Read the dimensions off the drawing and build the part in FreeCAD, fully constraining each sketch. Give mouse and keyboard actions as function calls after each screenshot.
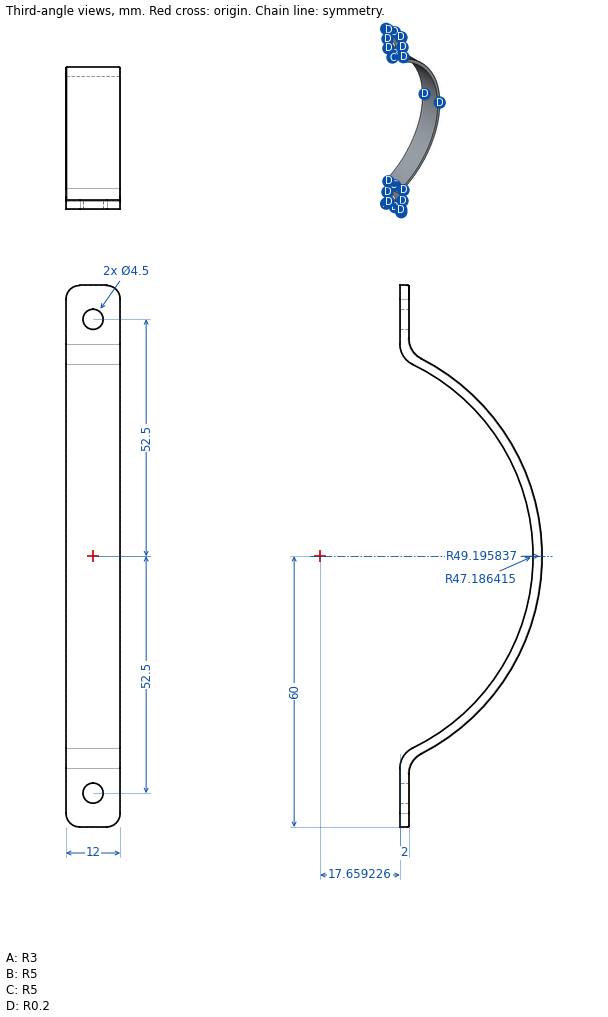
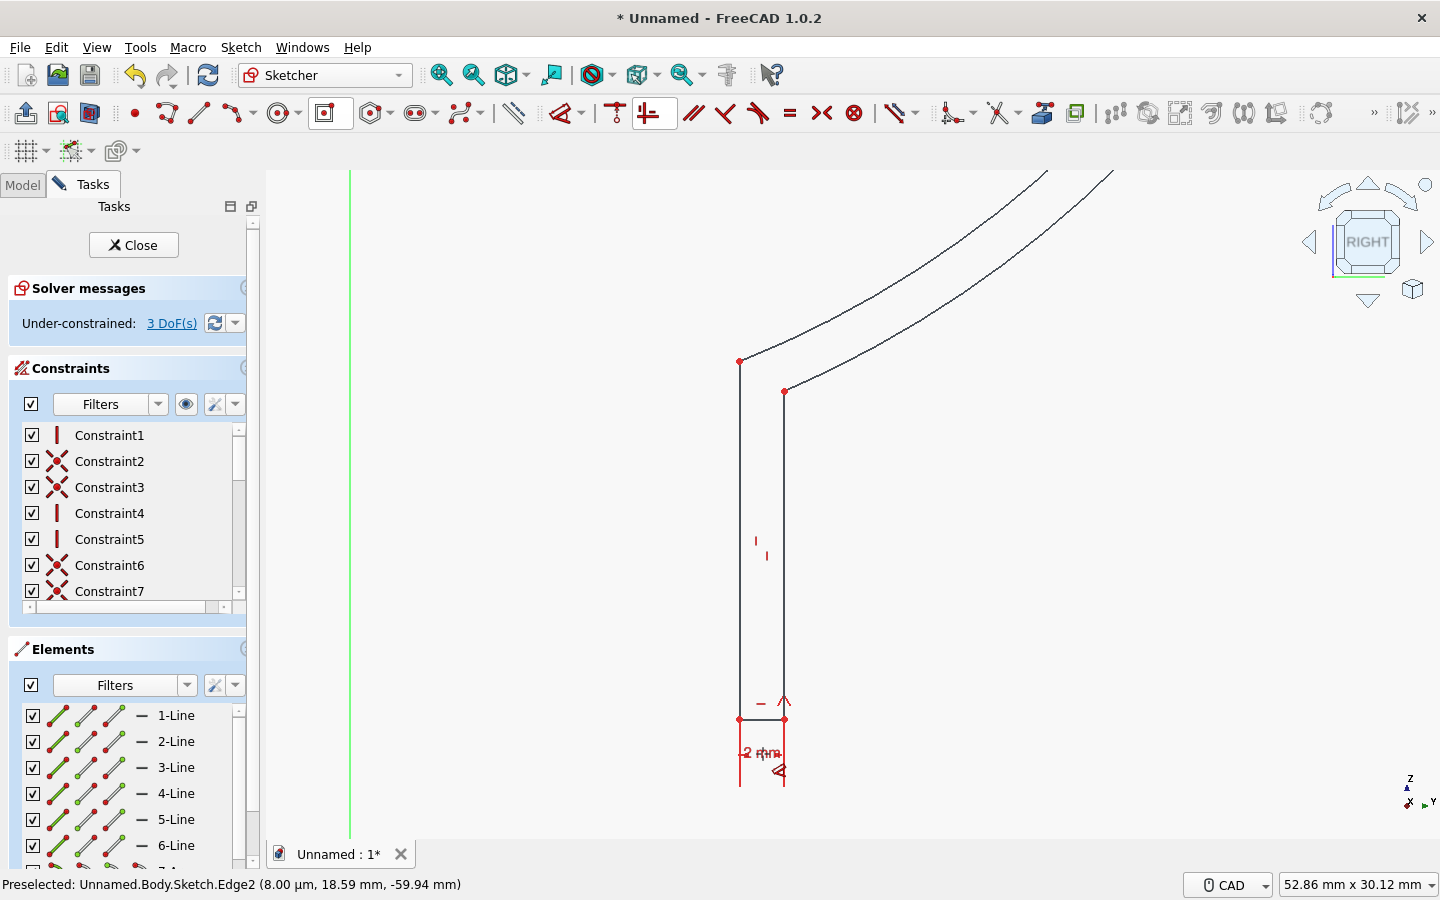
scroll(762, 725, down, 9)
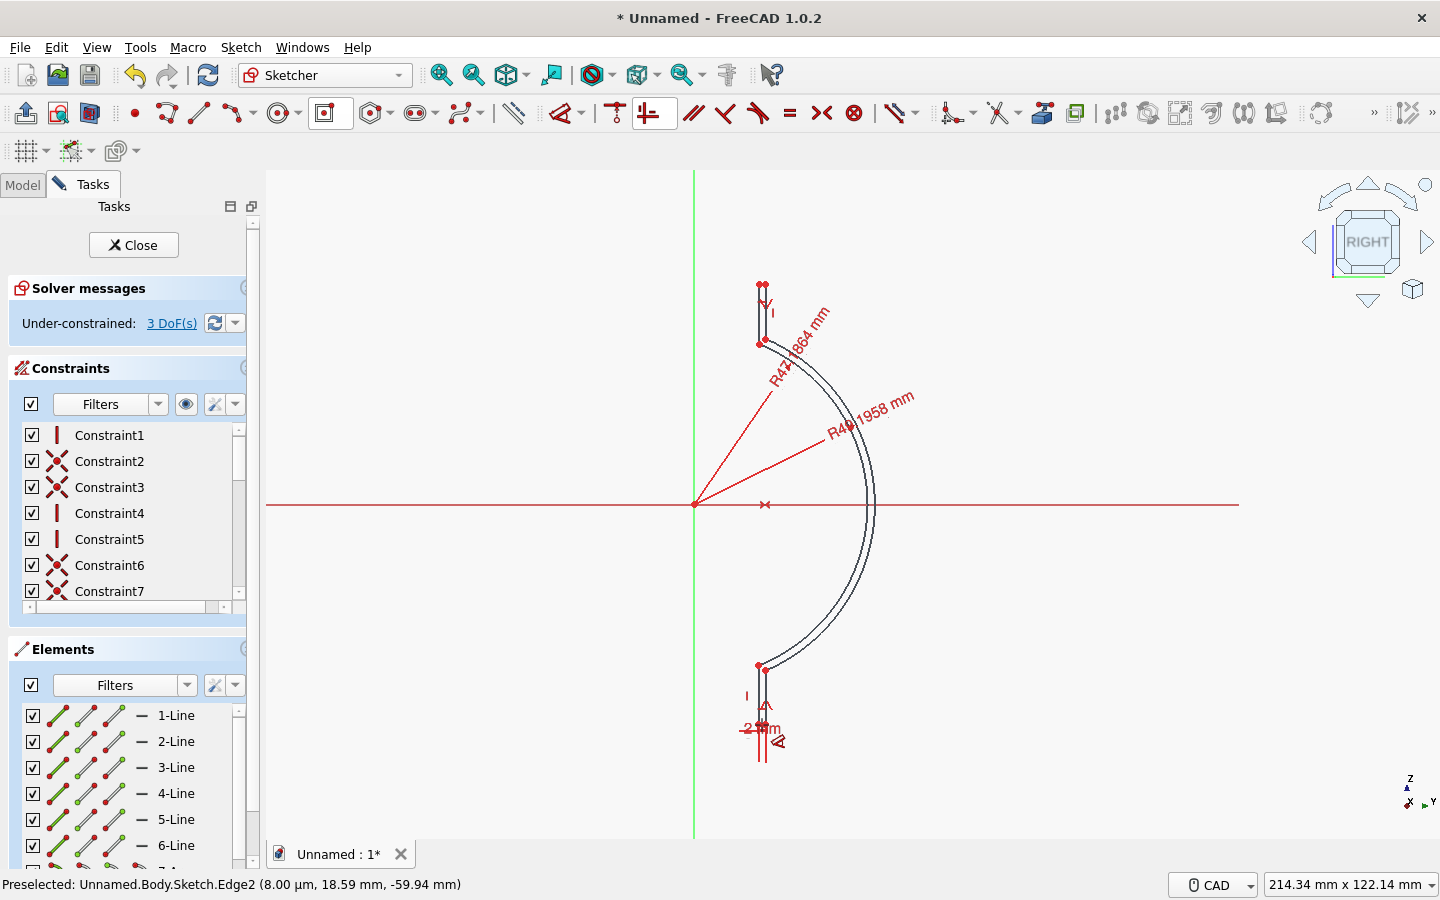
scroll(764, 285, up, 10)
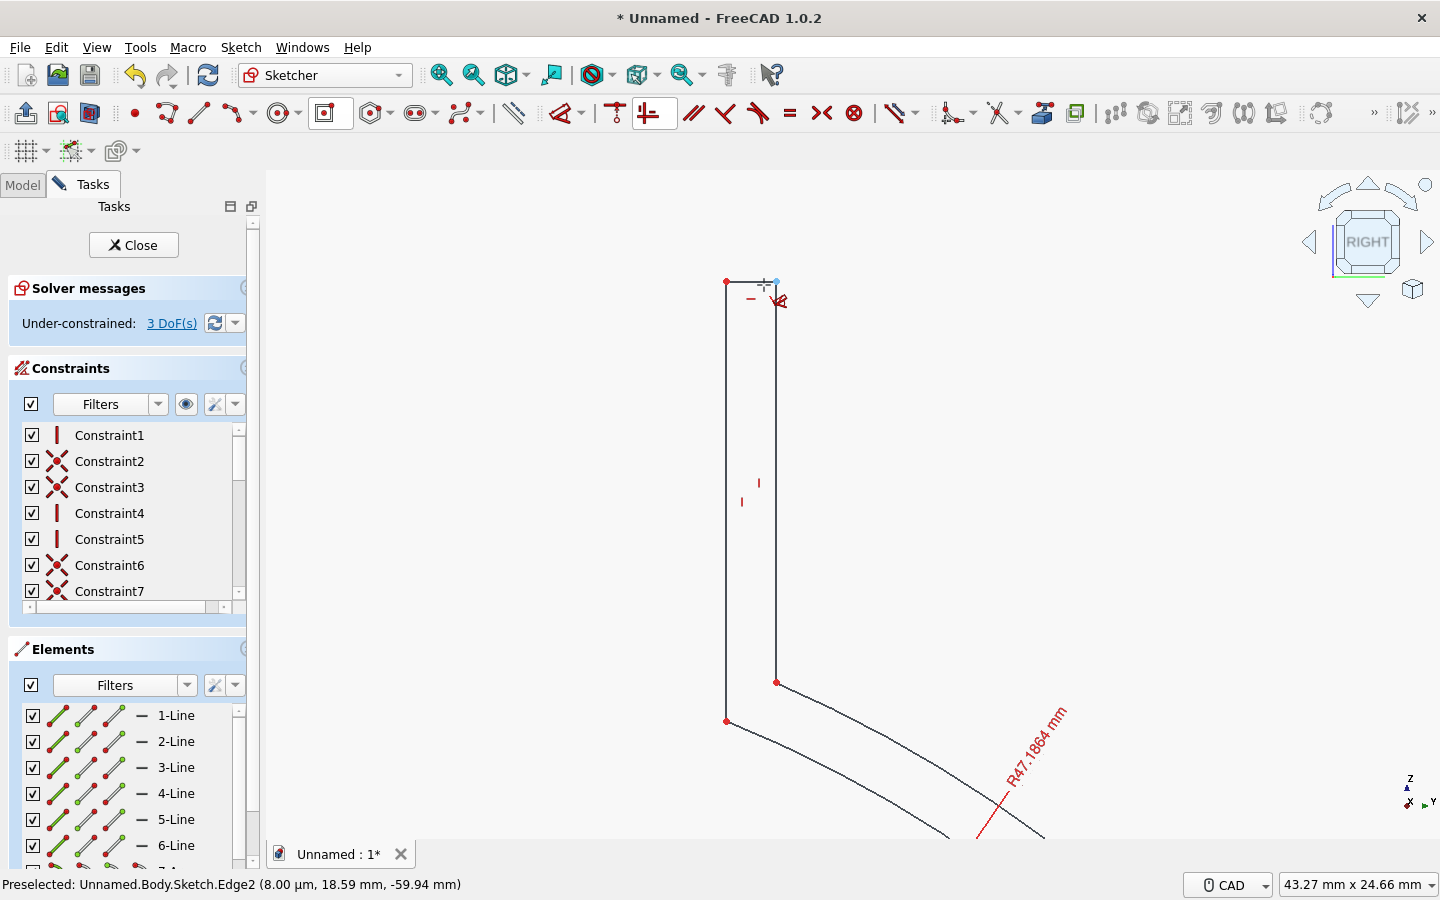
click(761, 282)
click(751, 248)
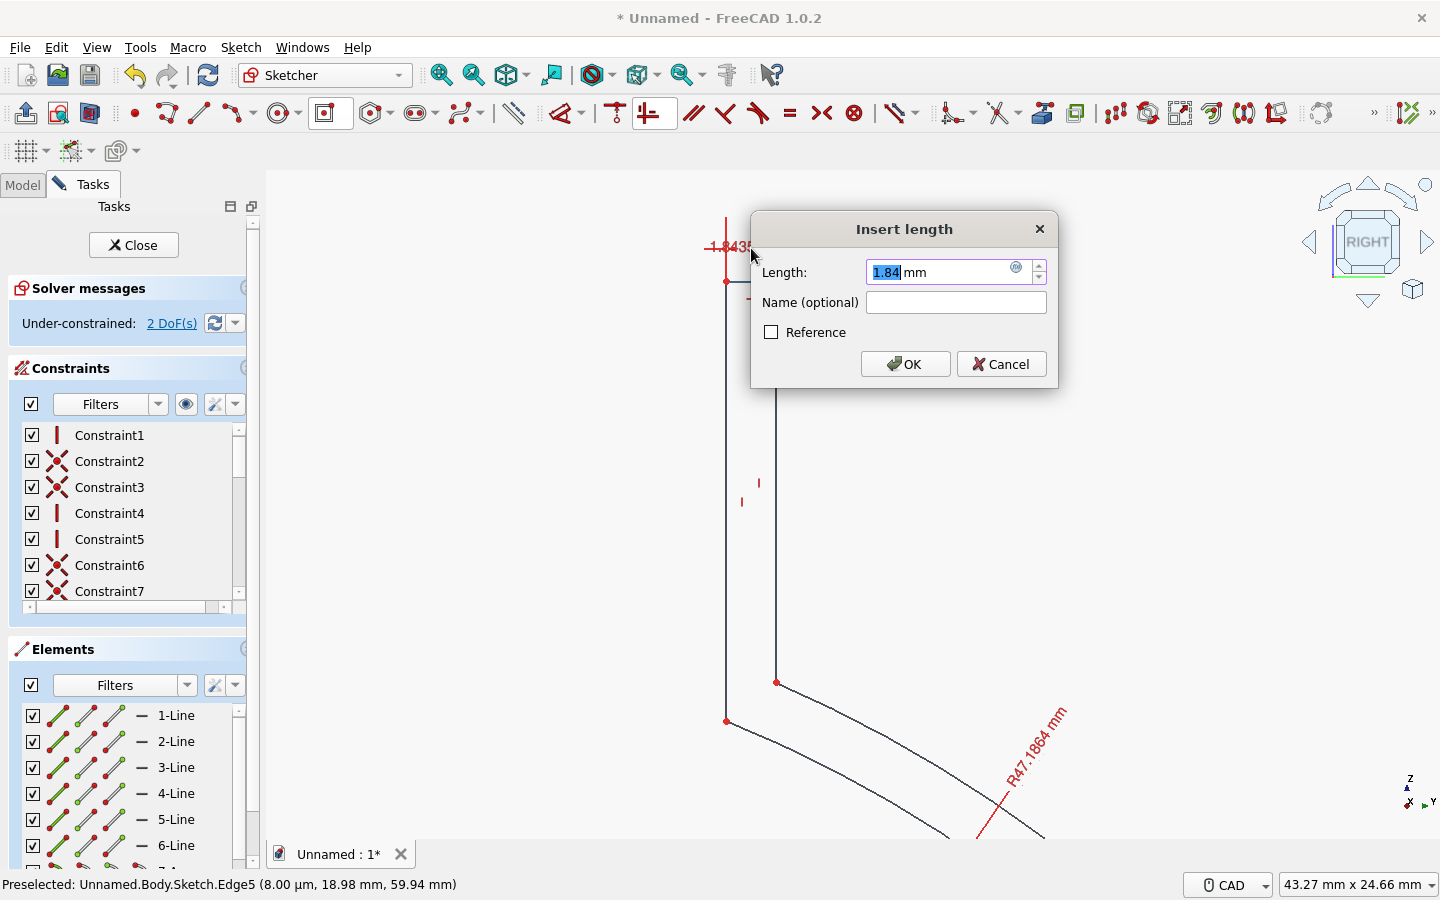
text(2)
key(Return)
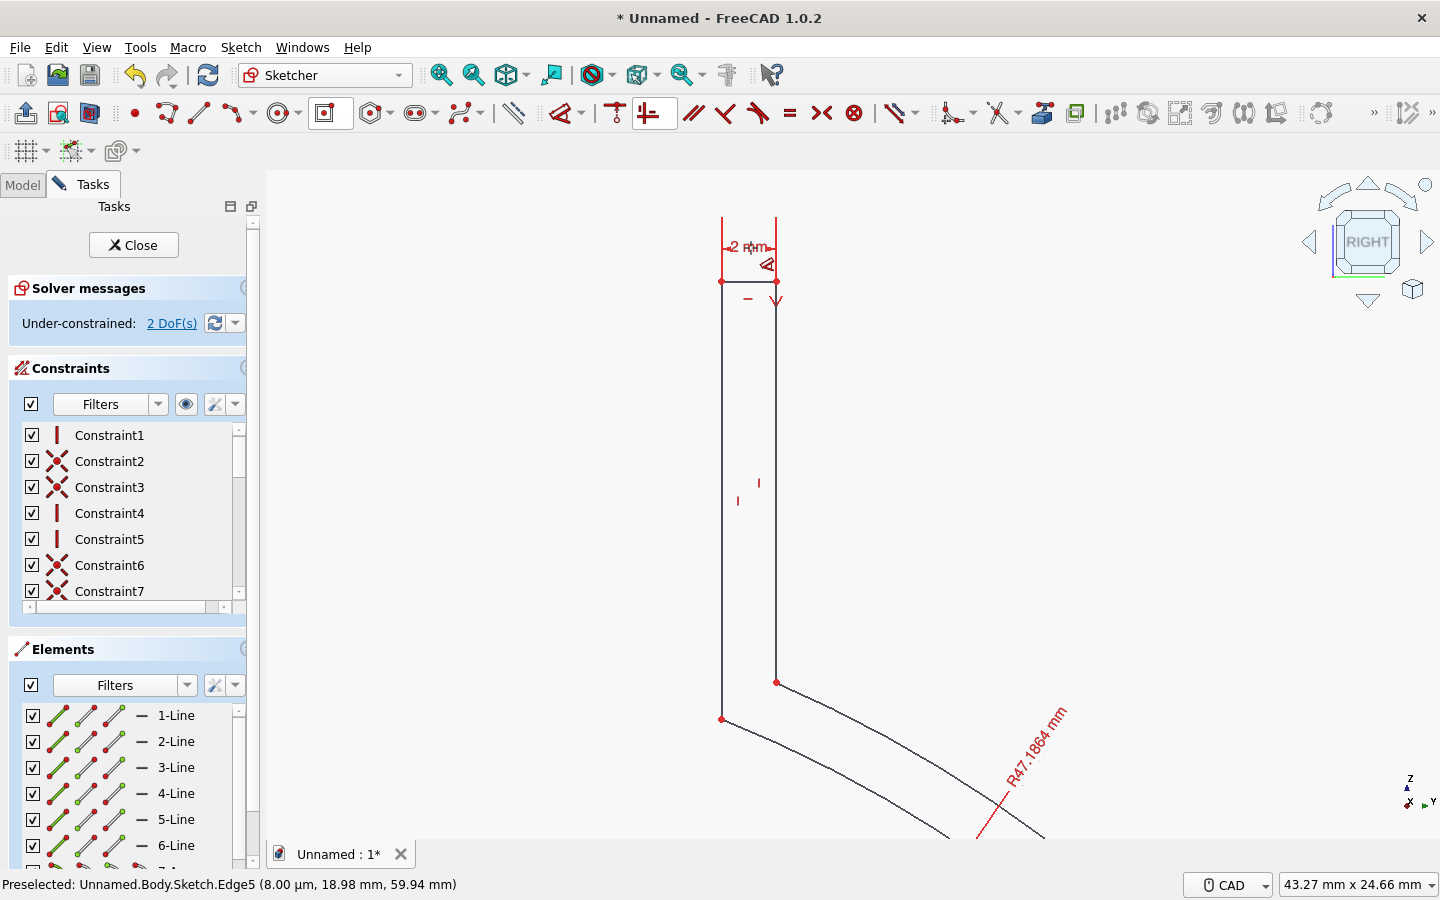
scroll(764, 285, down, 10)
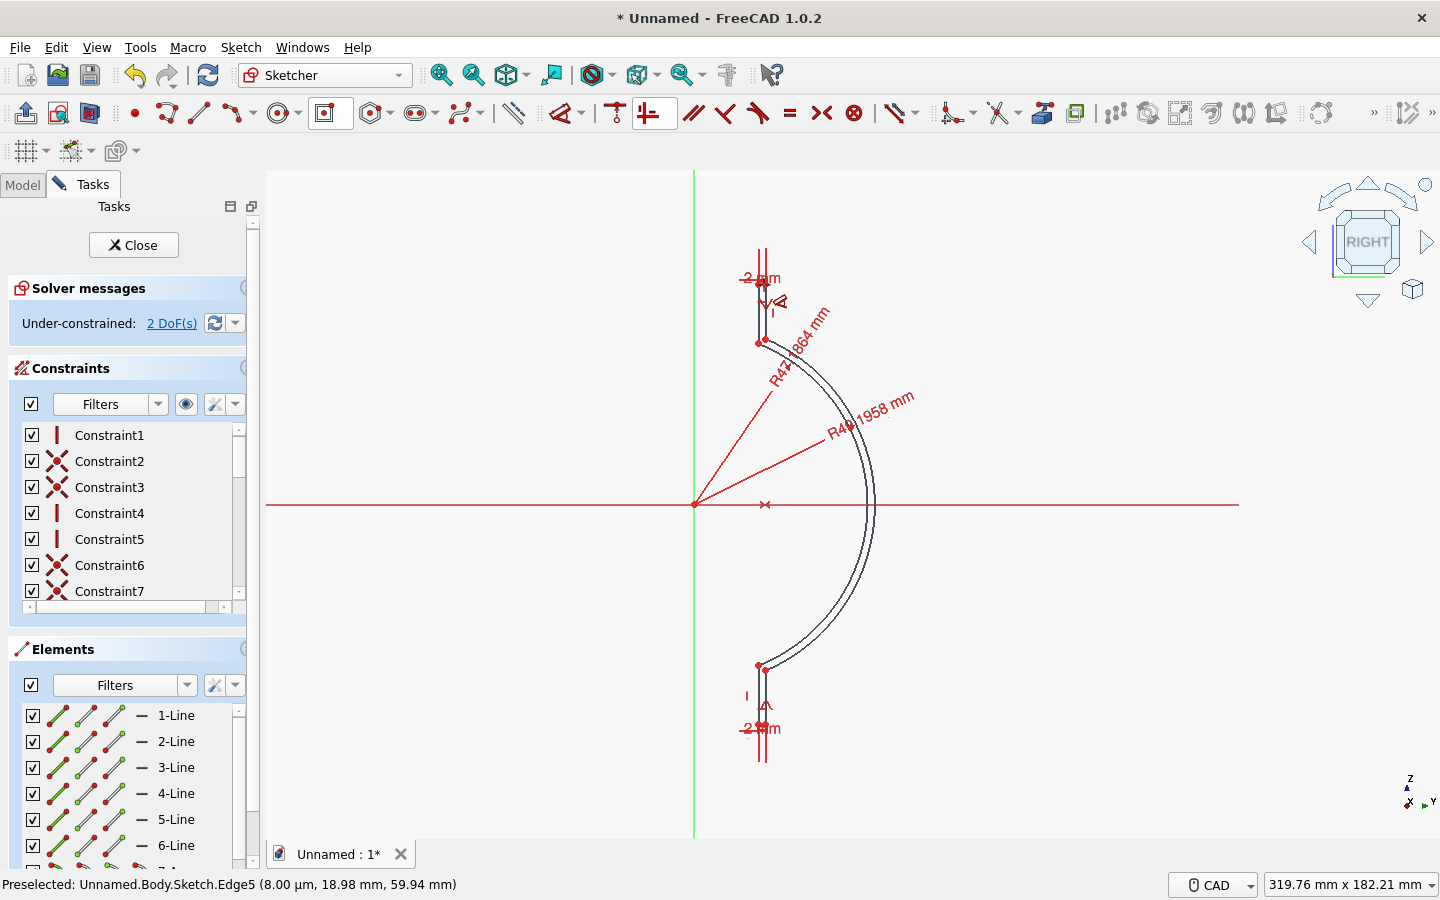
scroll(759, 725, up, 3)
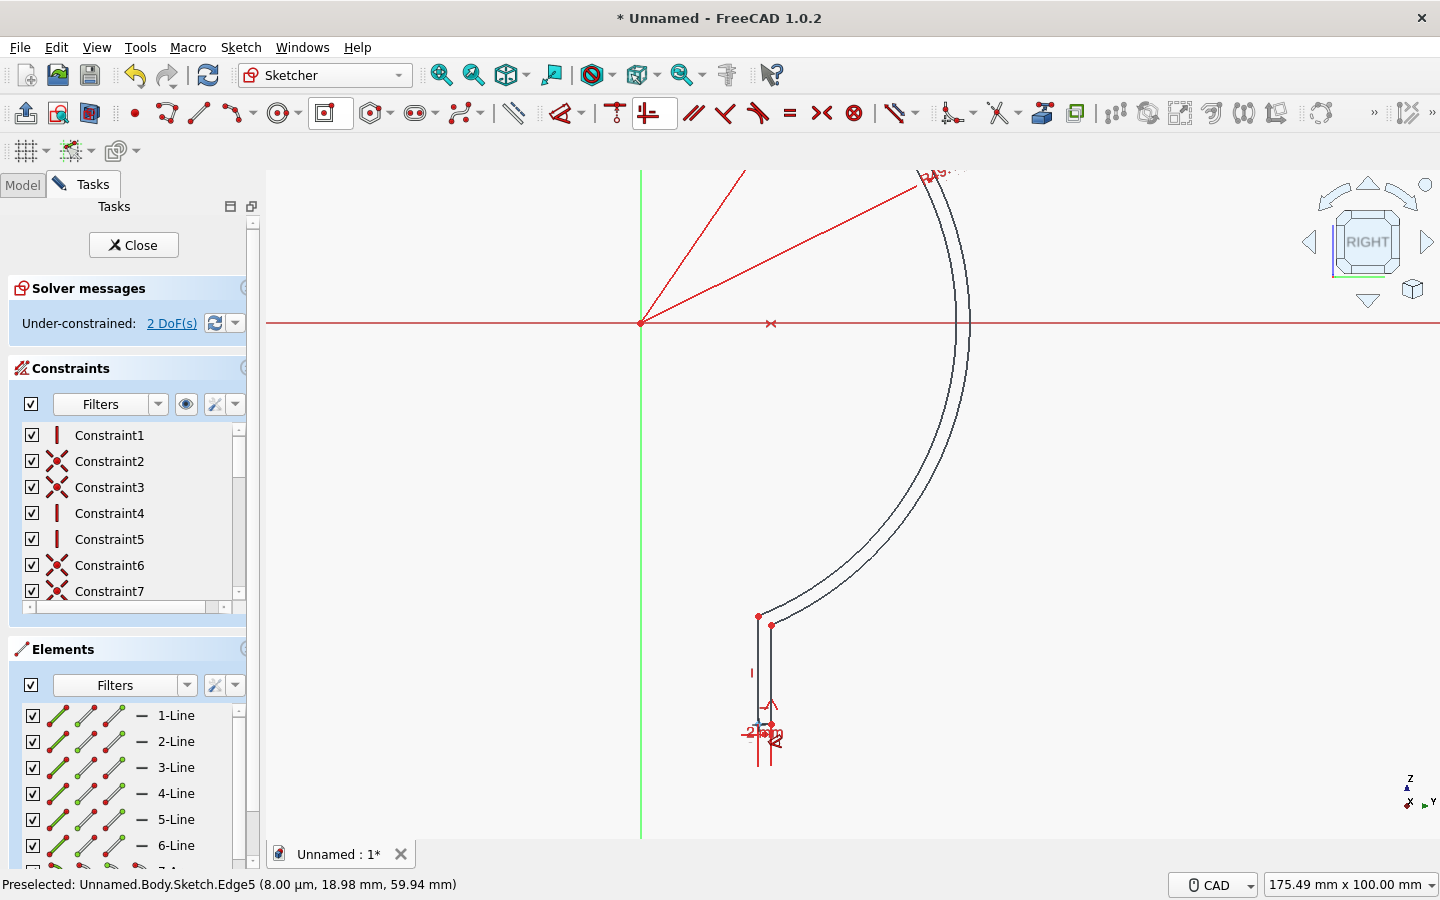
click(758, 724)
click(607, 524)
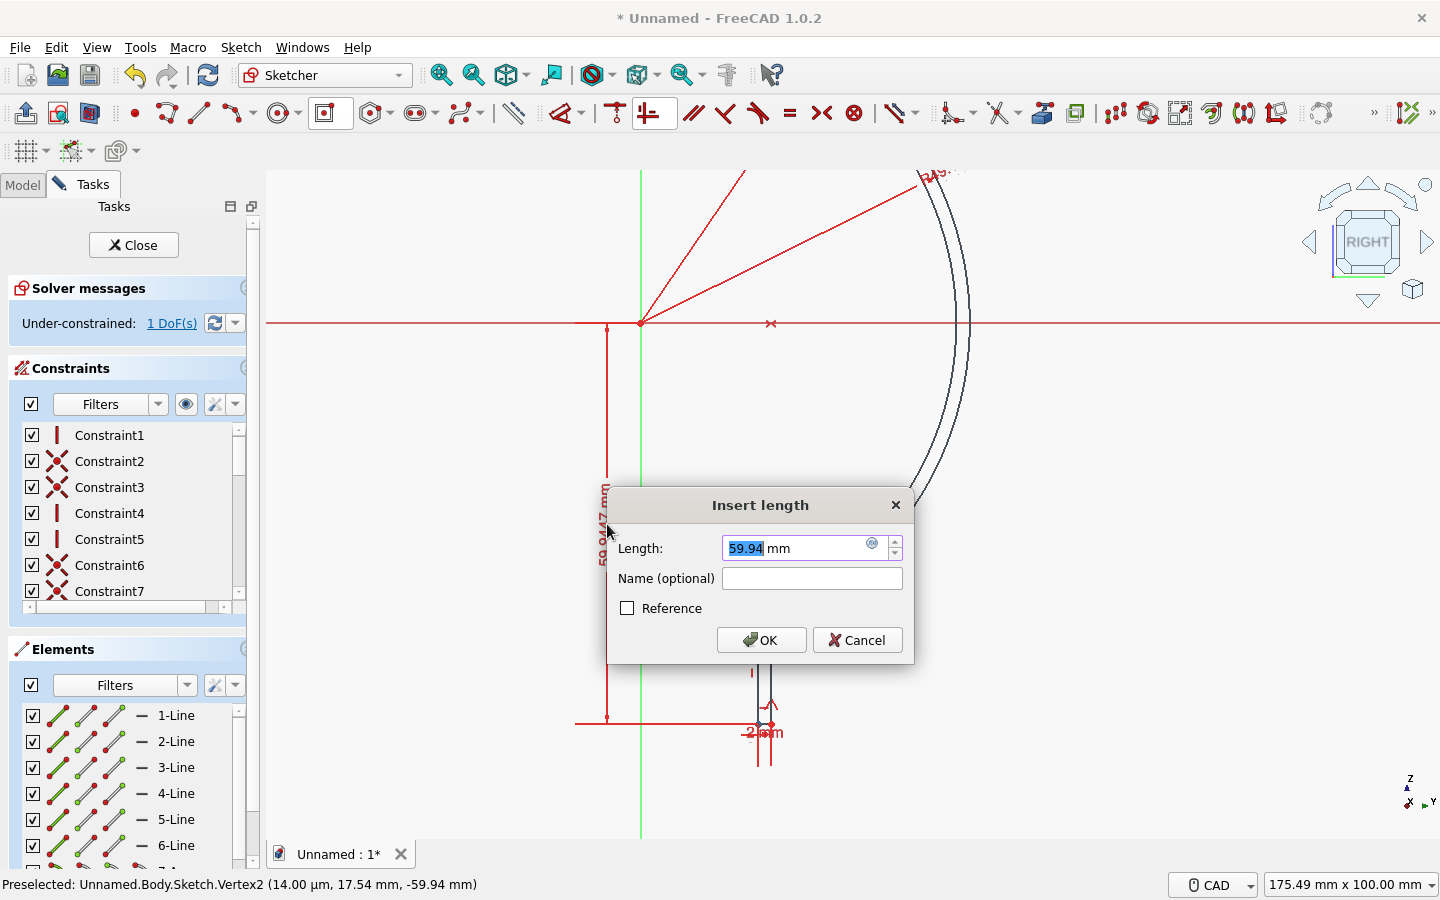
text(60)
key(Return)